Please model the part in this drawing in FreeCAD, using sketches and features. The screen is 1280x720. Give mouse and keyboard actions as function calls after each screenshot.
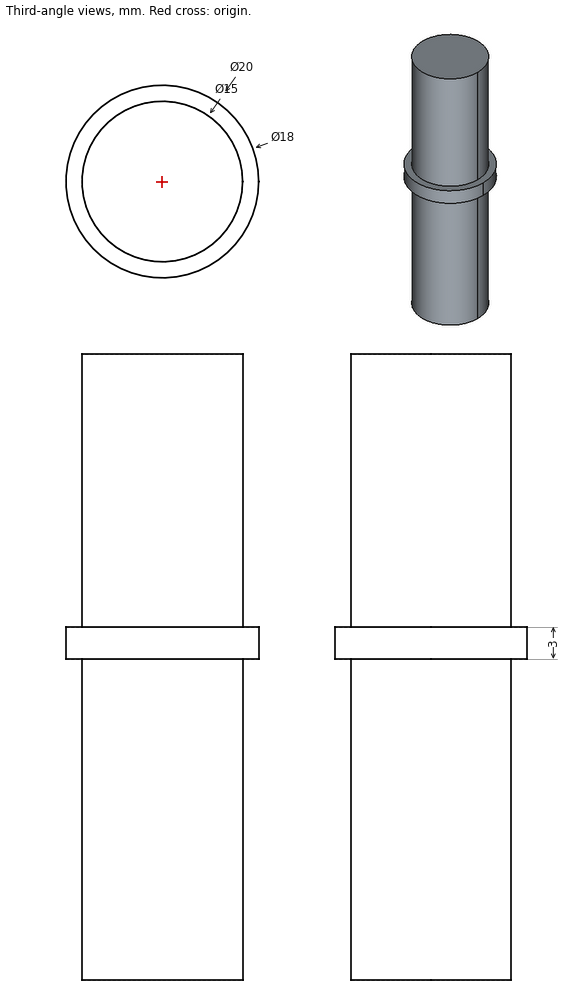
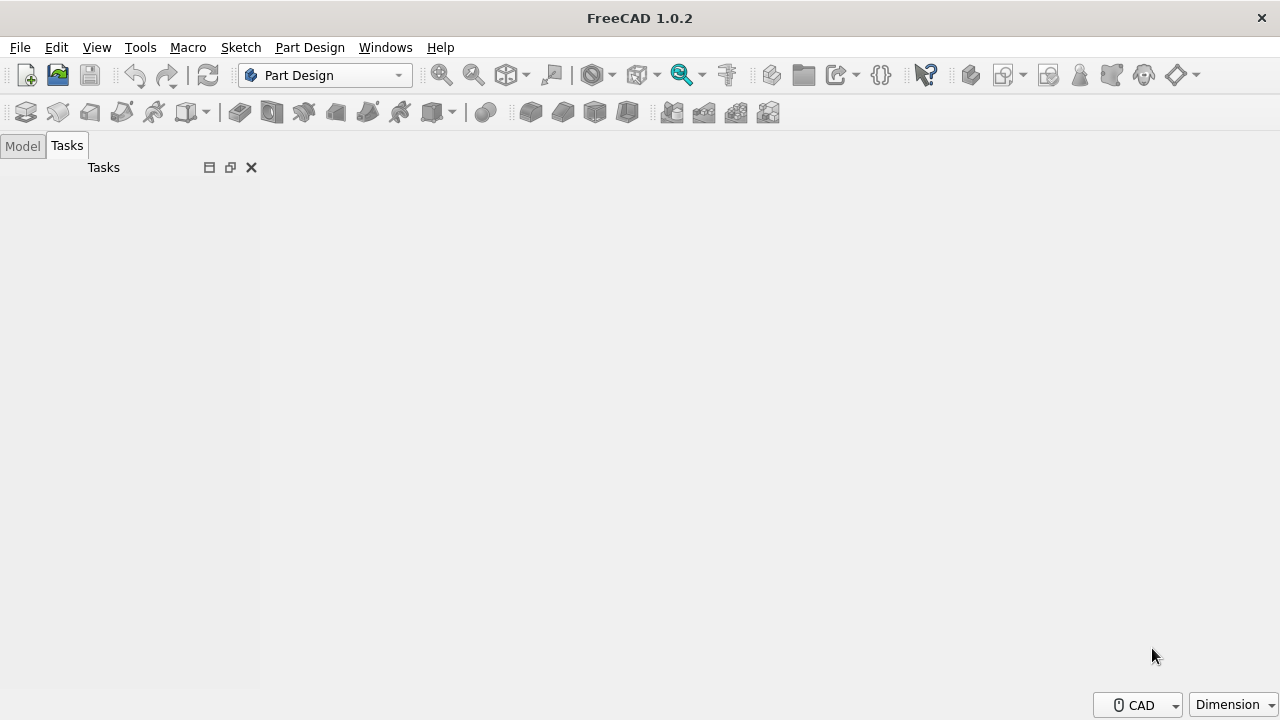
click(26, 76)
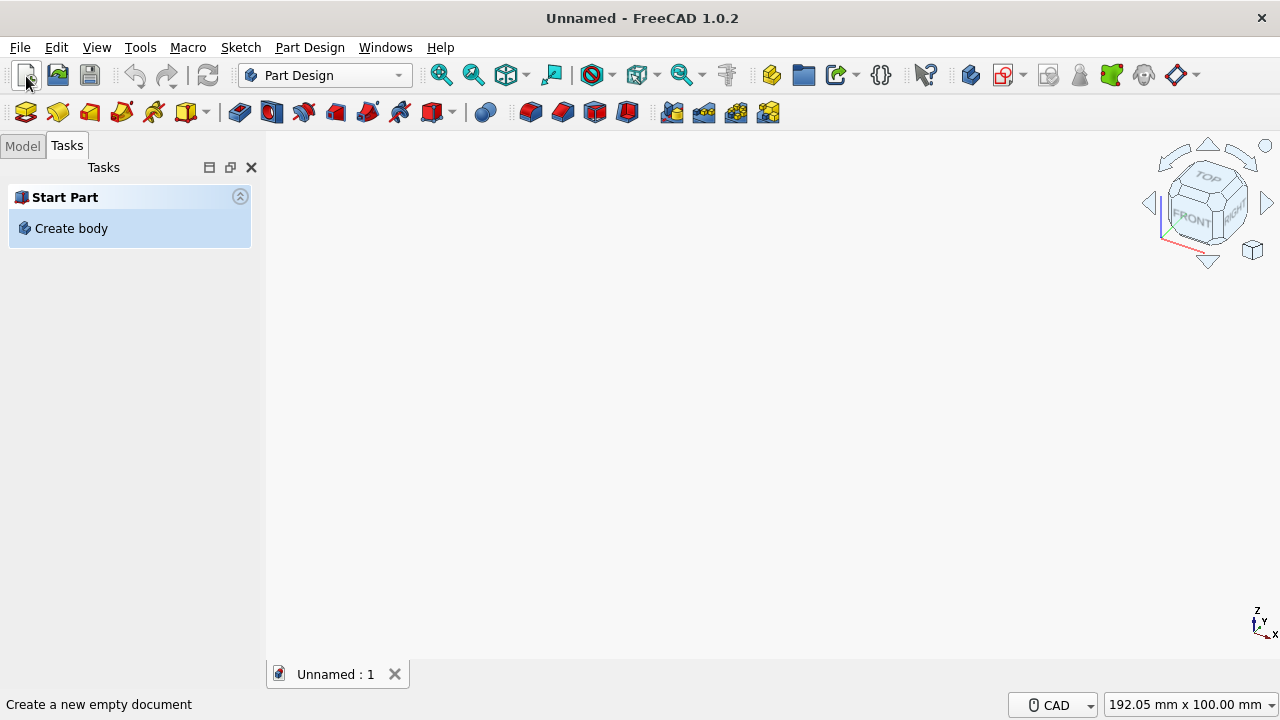
click(1004, 76)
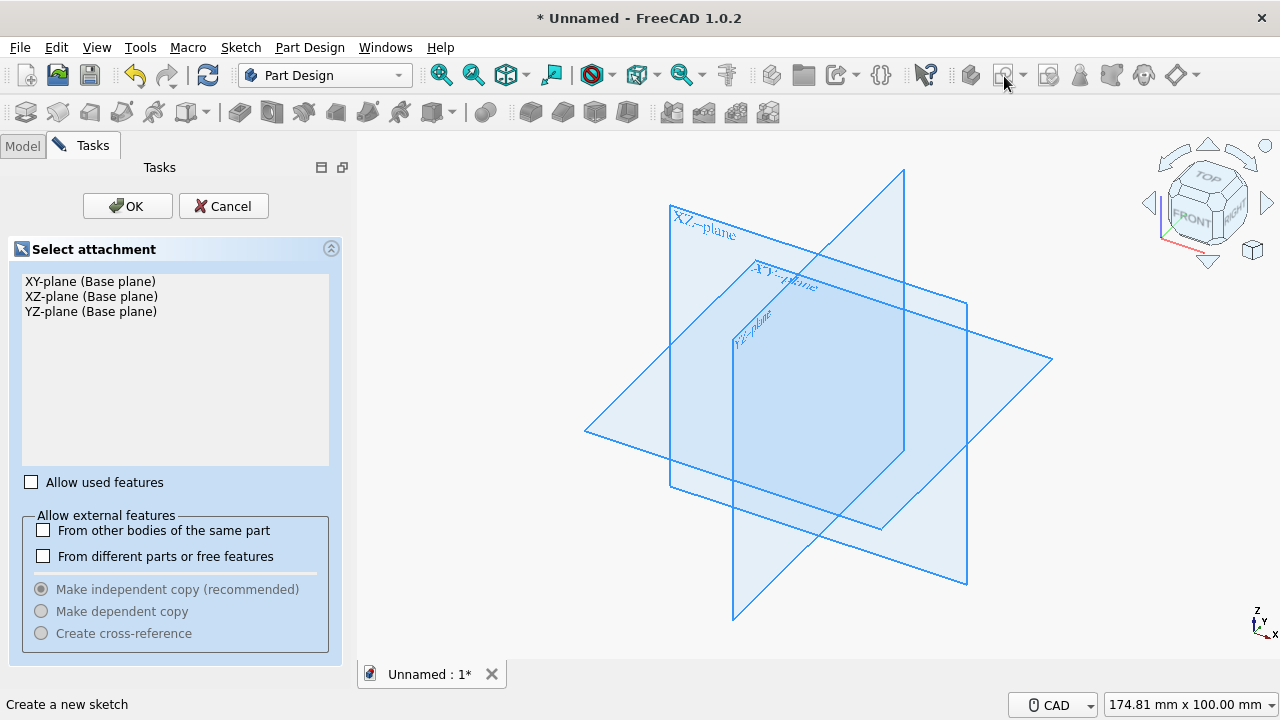
click(82, 282)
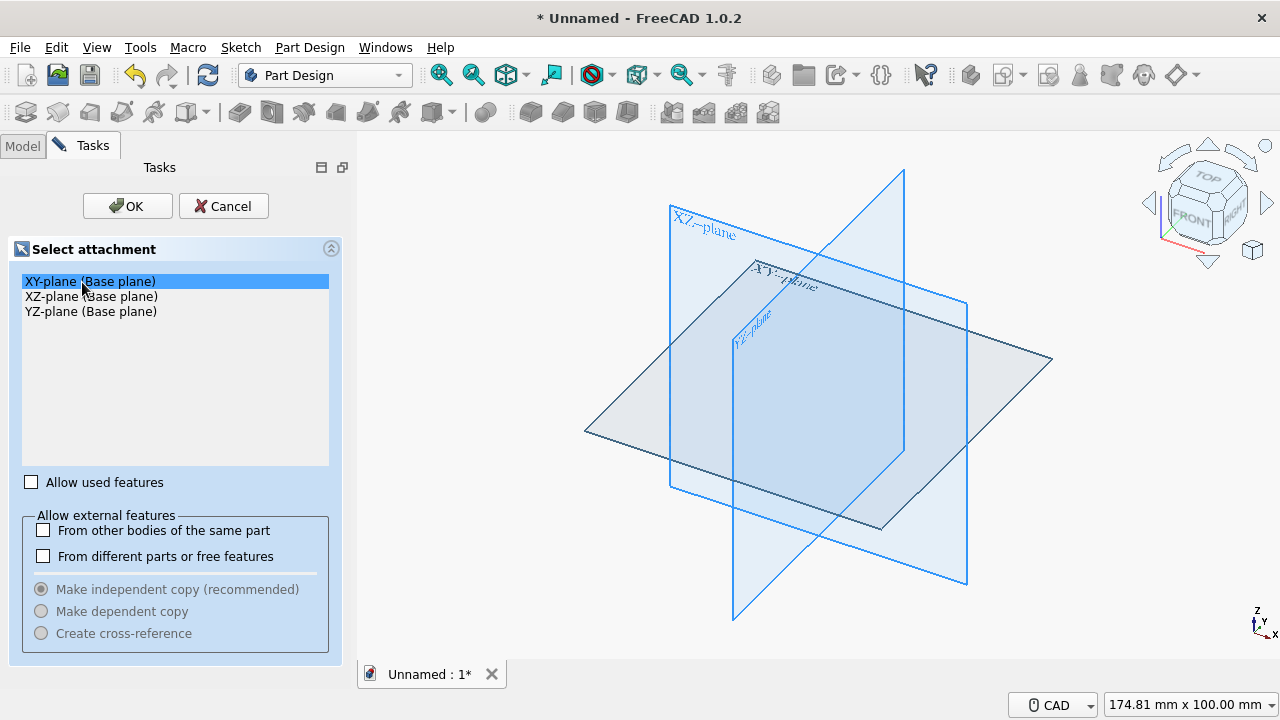
click(128, 206)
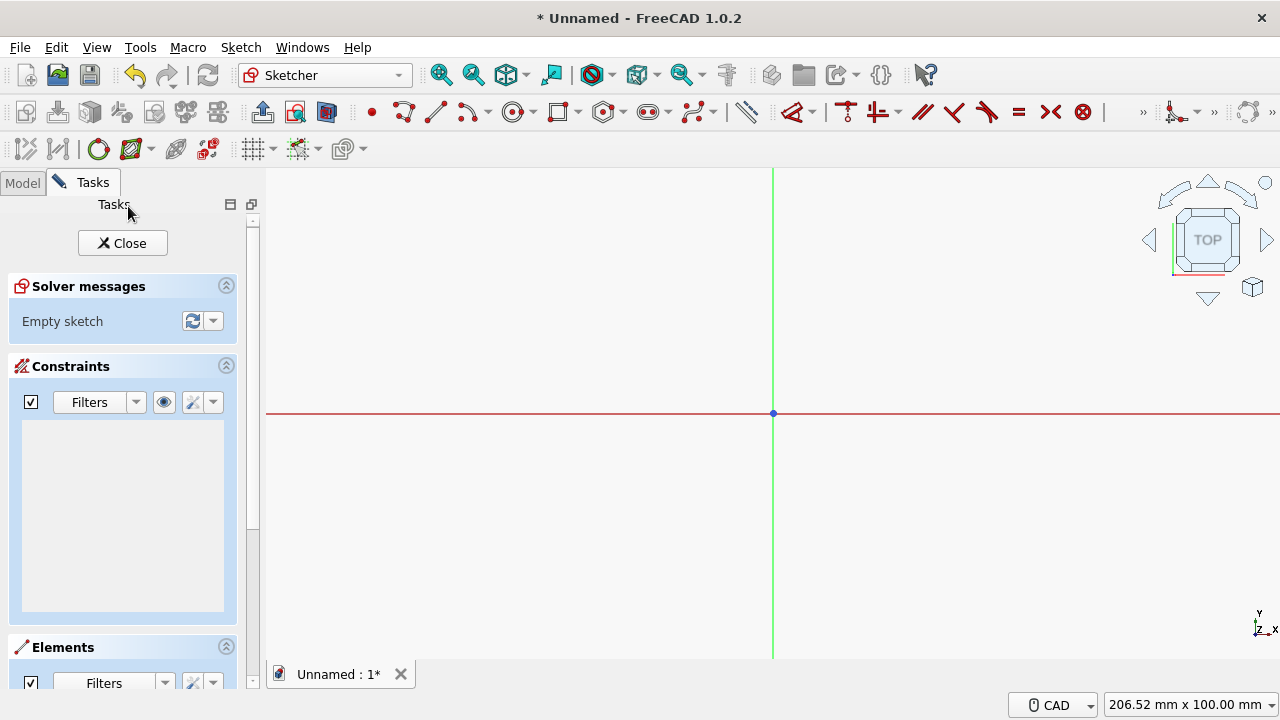
scroll(795, 414, up, 7)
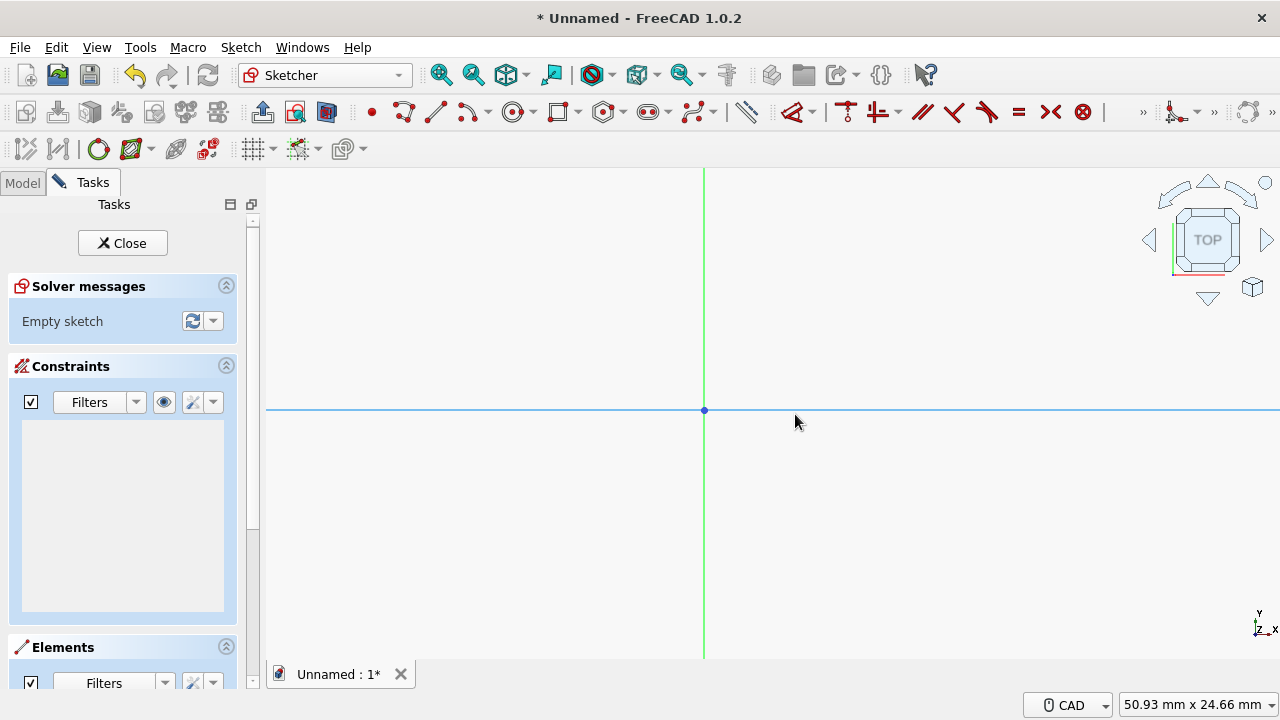
click(514, 112)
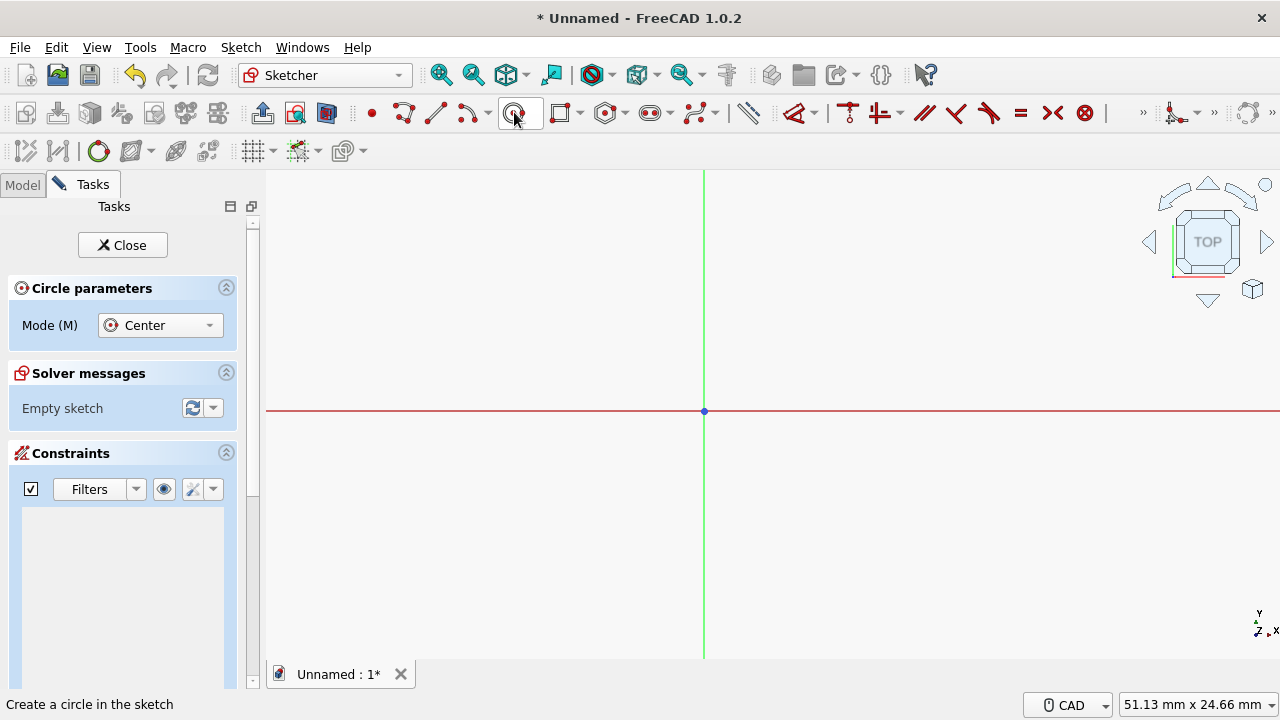
click(704, 411)
click(810, 306)
key(Escape)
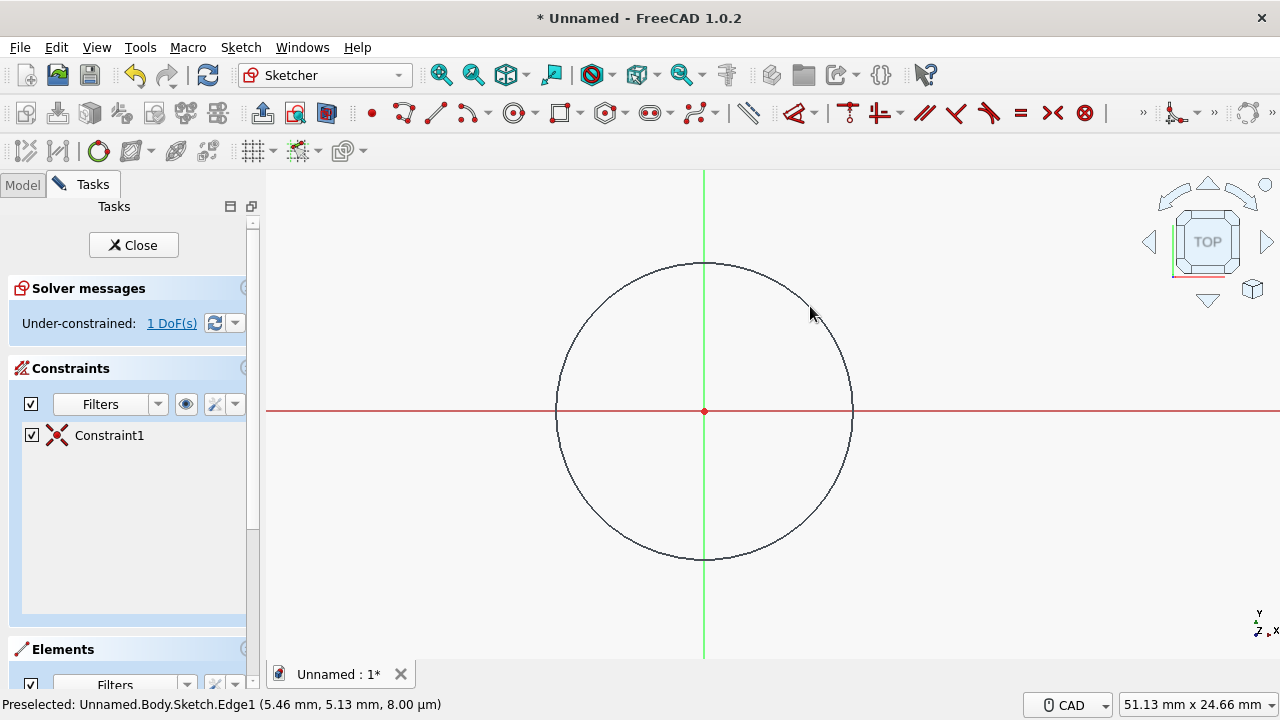
click(794, 114)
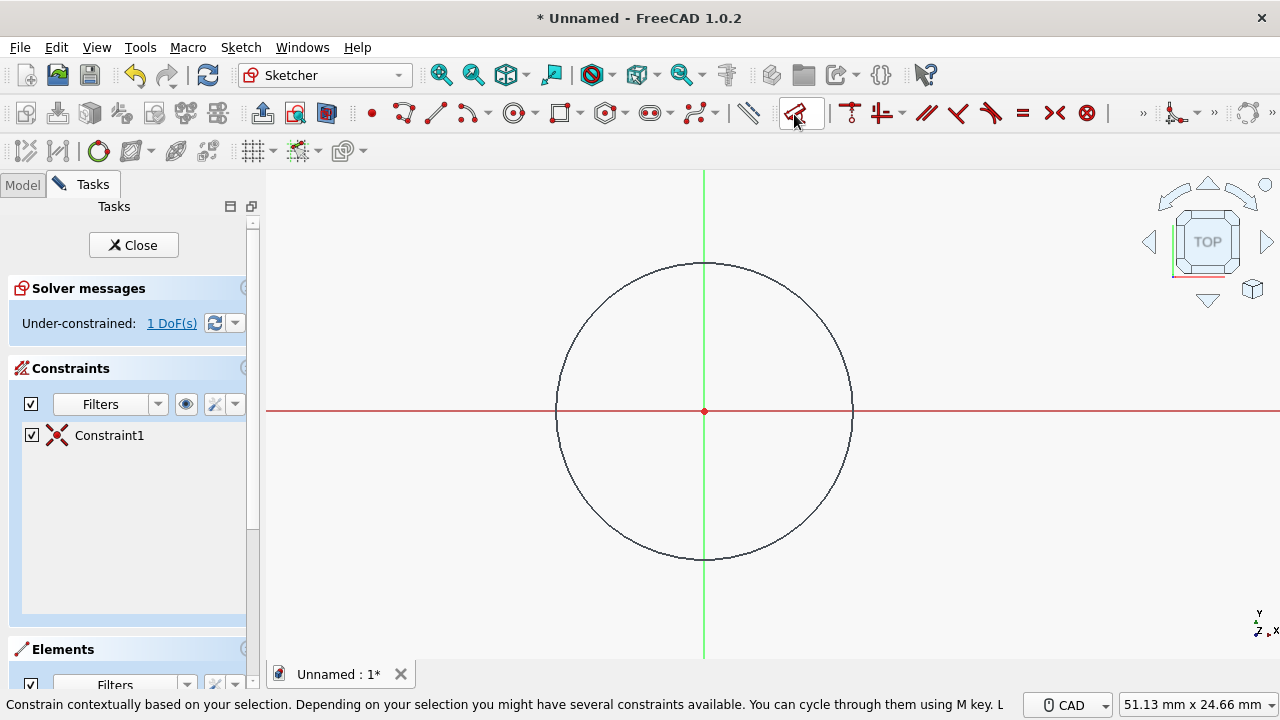
click(809, 306)
click(832, 283)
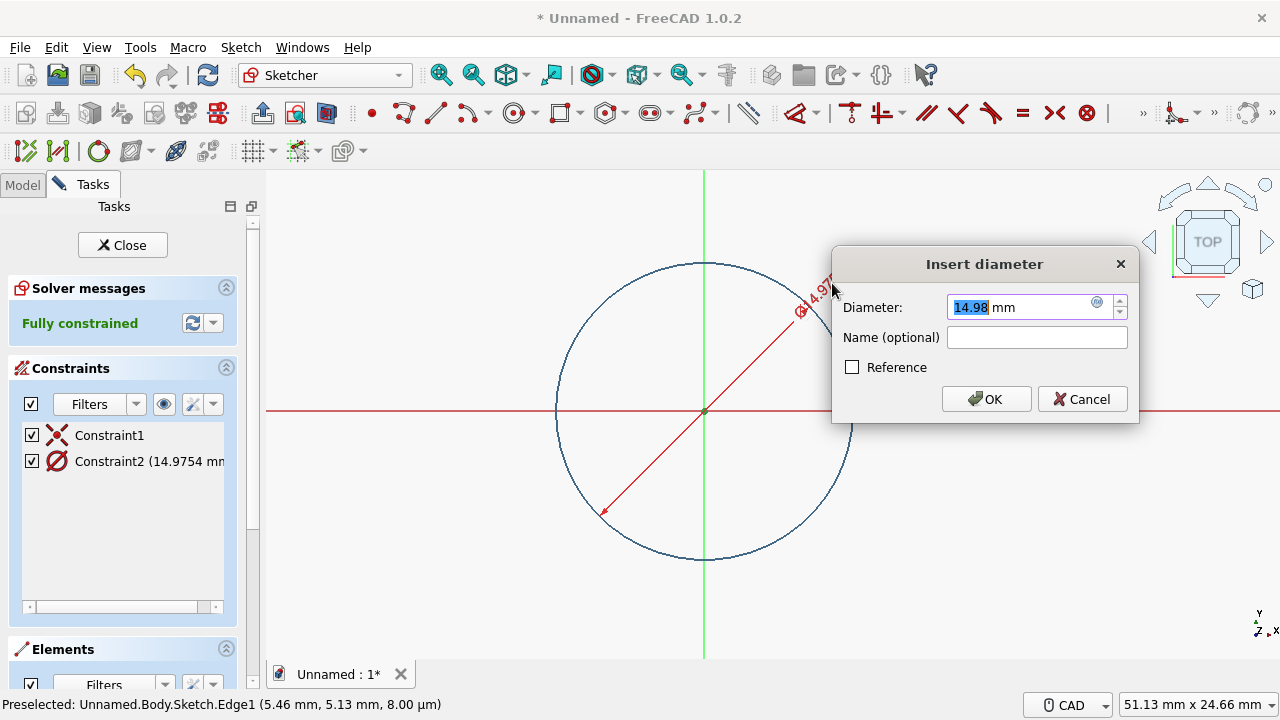
text(15)
key(Return)
key(Escape)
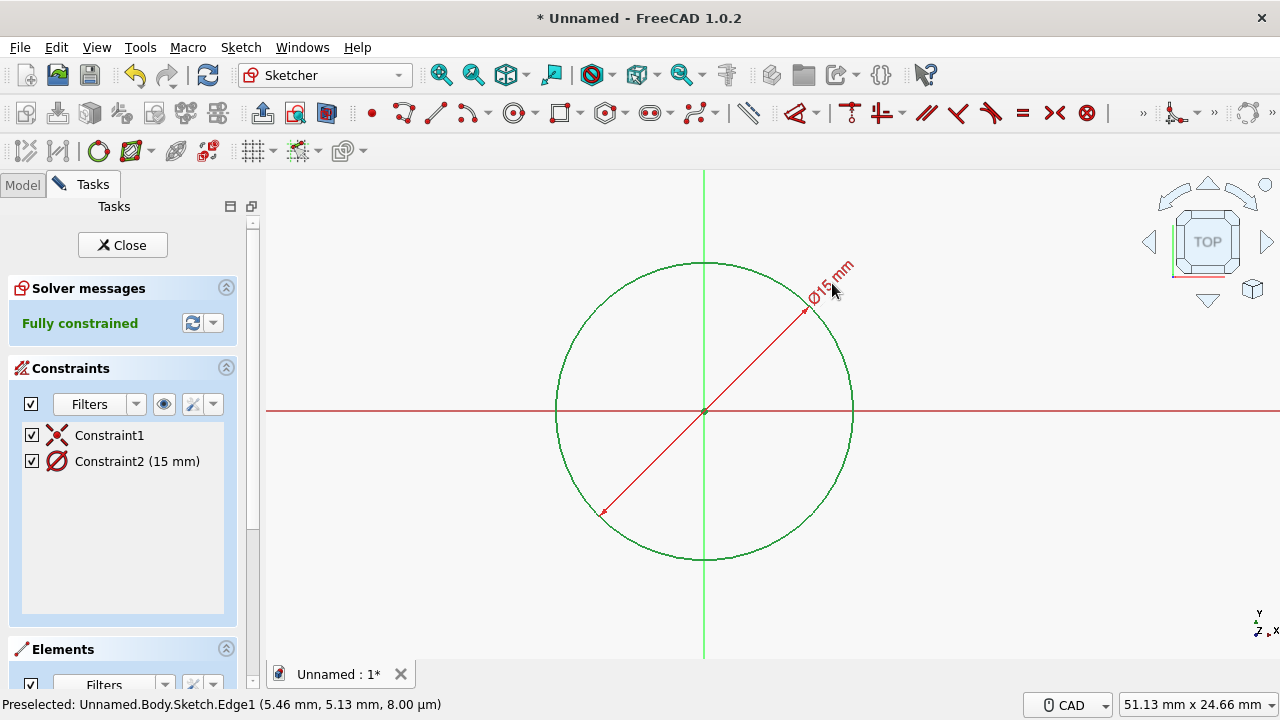
click(123, 245)